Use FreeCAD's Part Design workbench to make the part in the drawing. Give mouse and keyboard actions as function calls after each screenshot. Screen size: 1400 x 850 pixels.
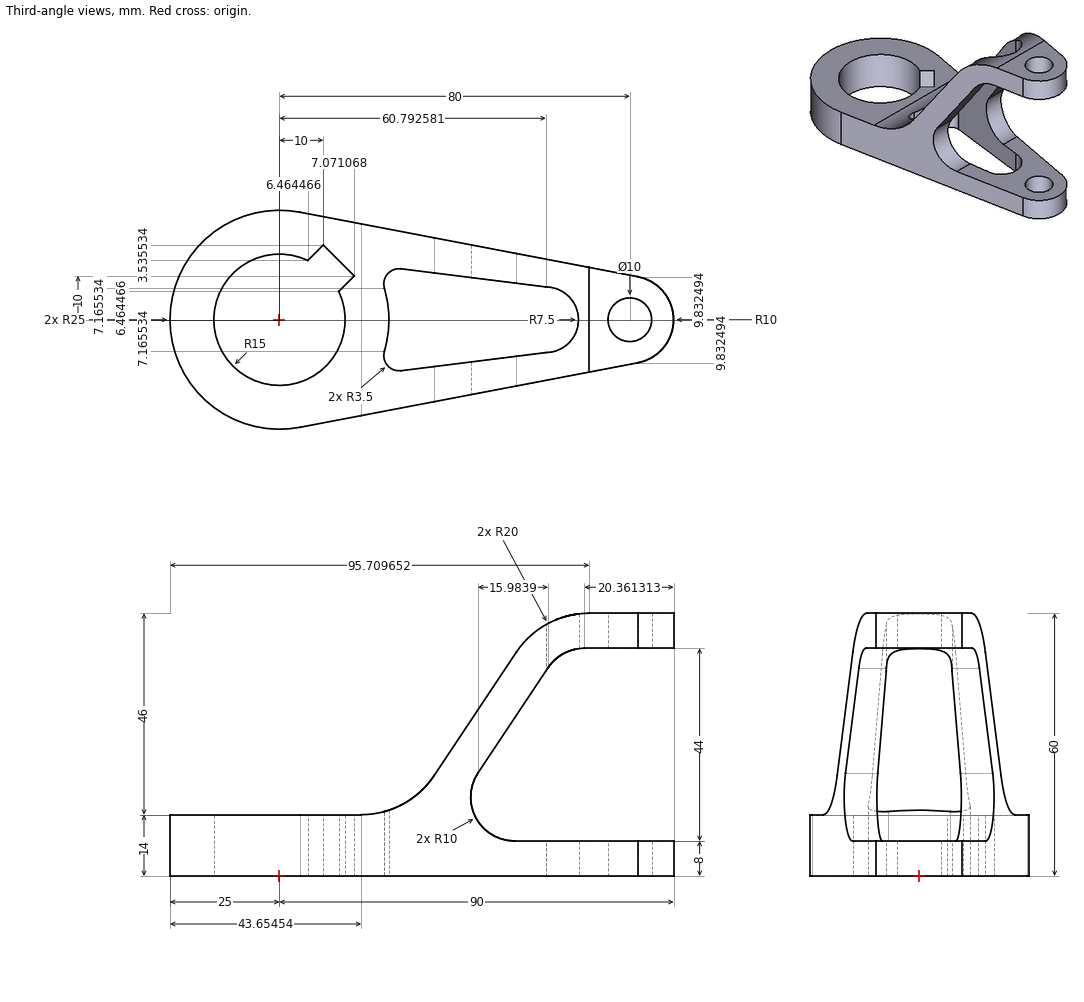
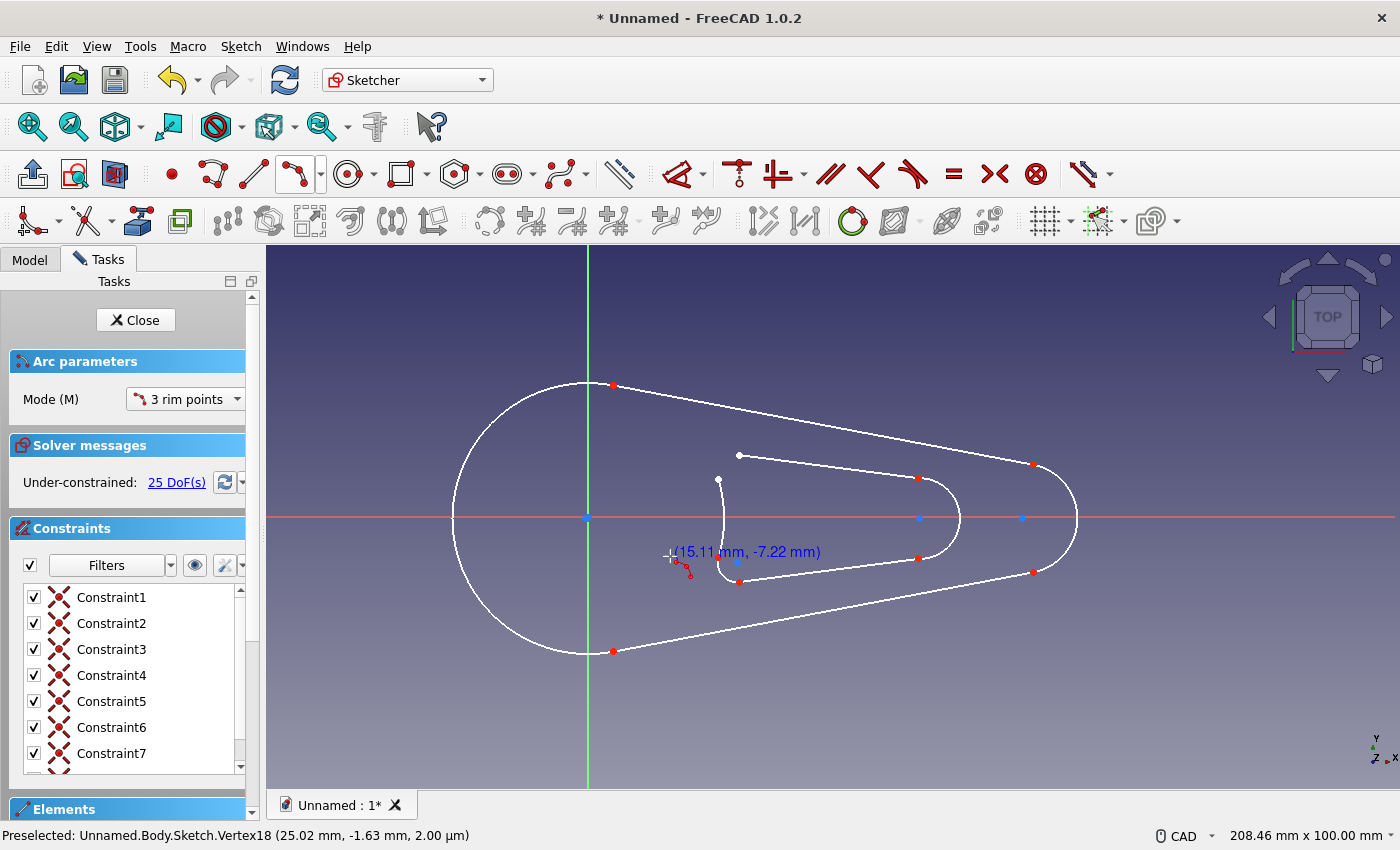
click(718, 479)
click(739, 455)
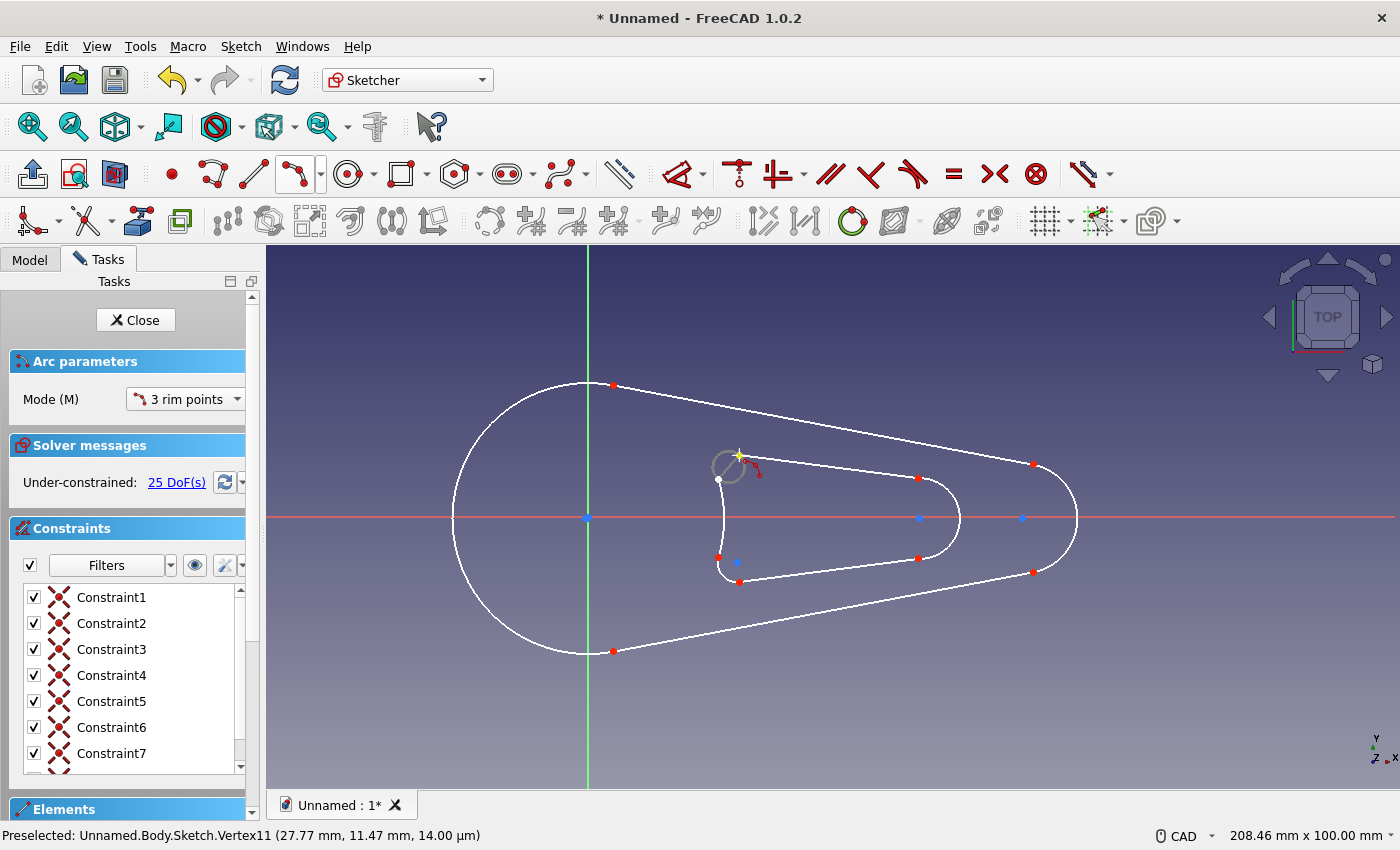
scroll(722, 461, up, 4)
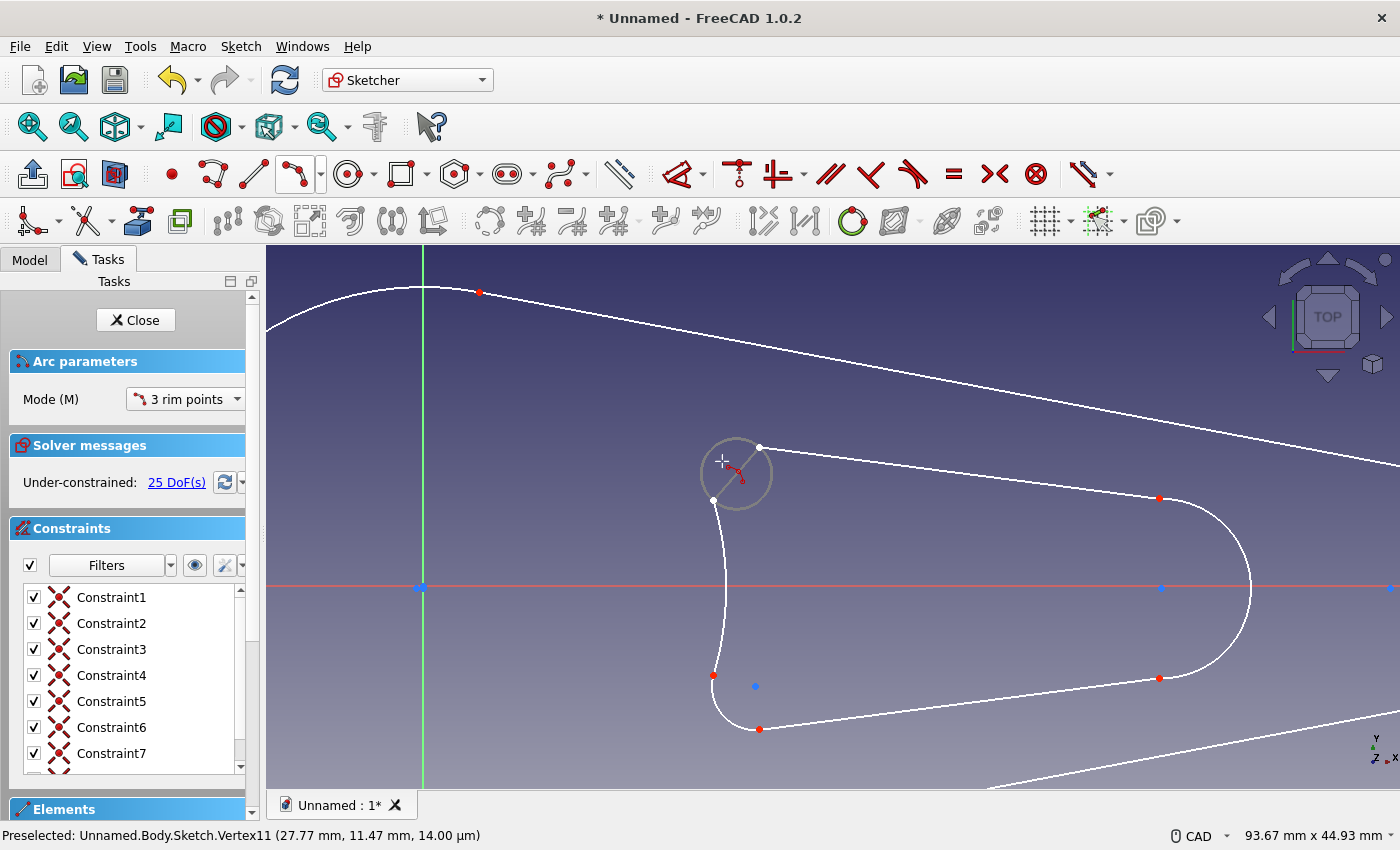
click(722, 460)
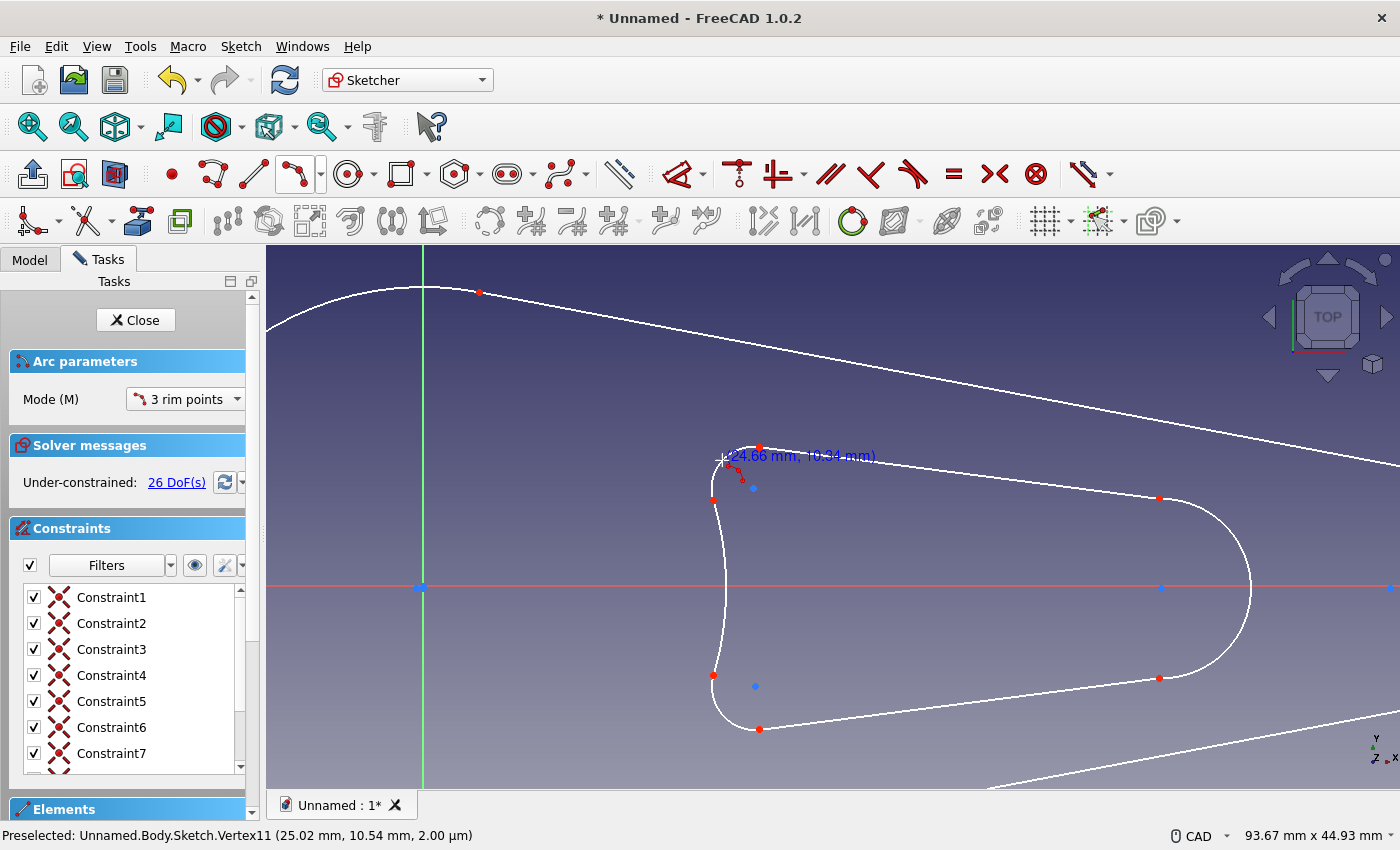
click(213, 174)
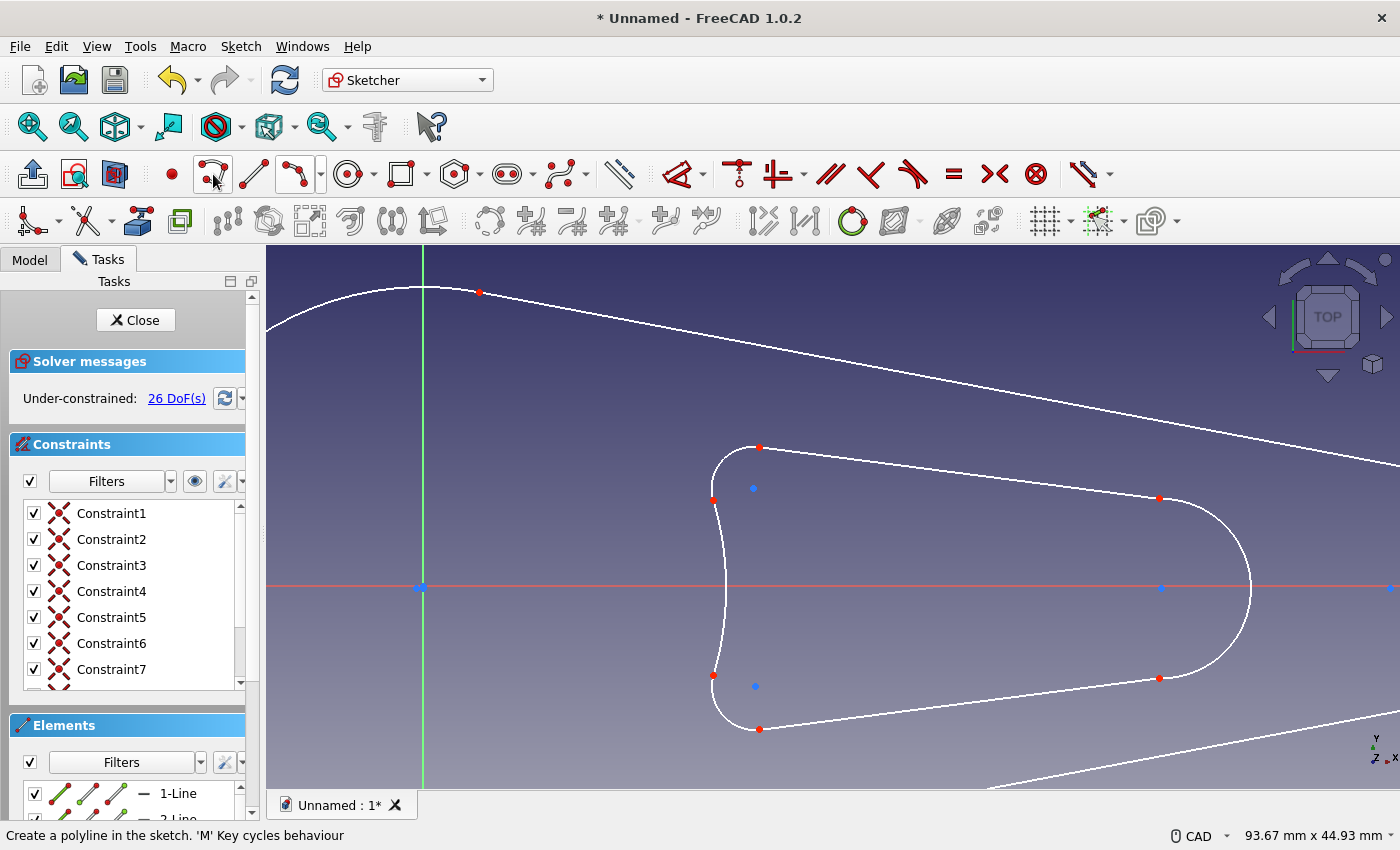
click(502, 422)
click(544, 379)
click(630, 465)
click(587, 508)
right_click(587, 508)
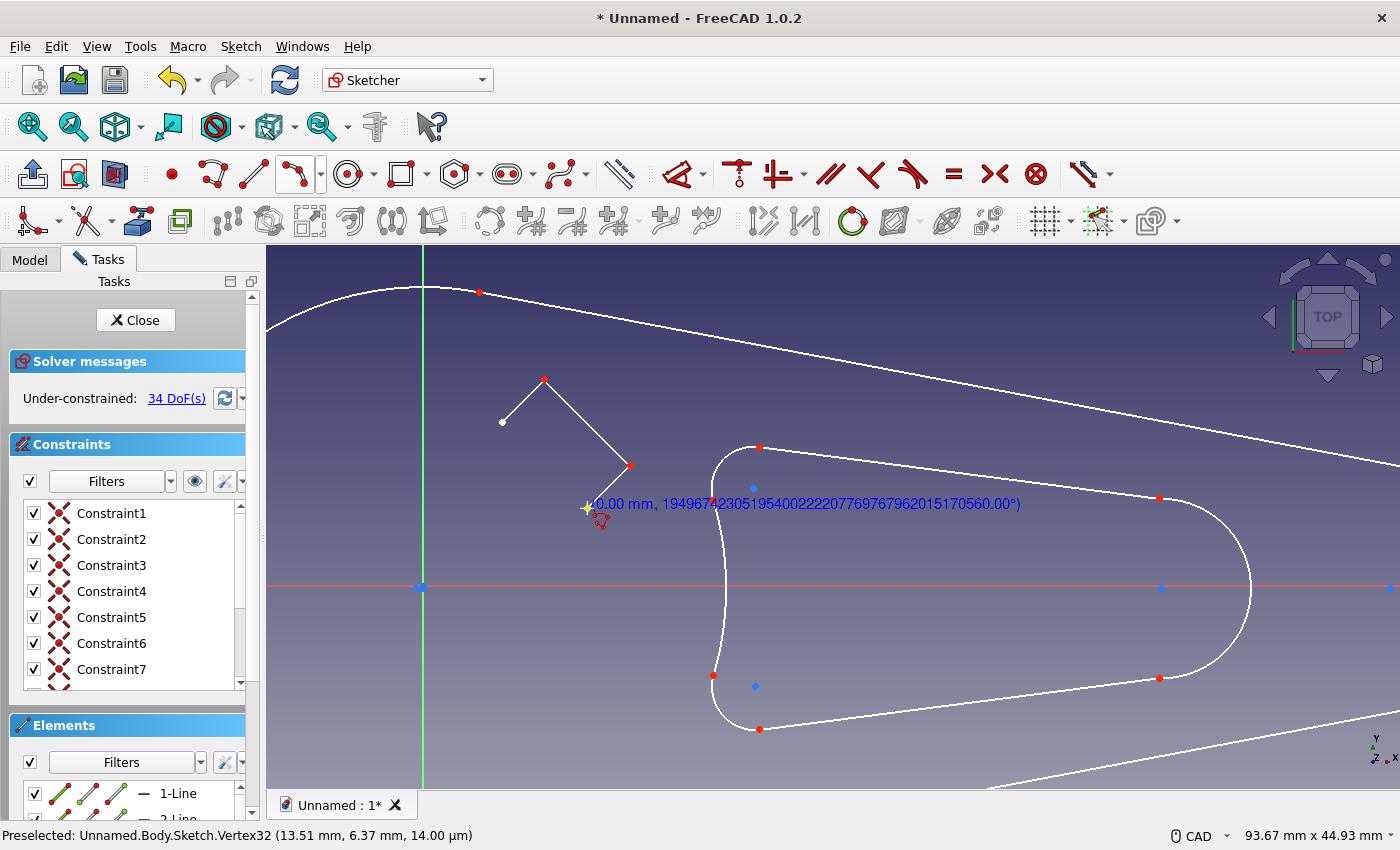
click(294, 174)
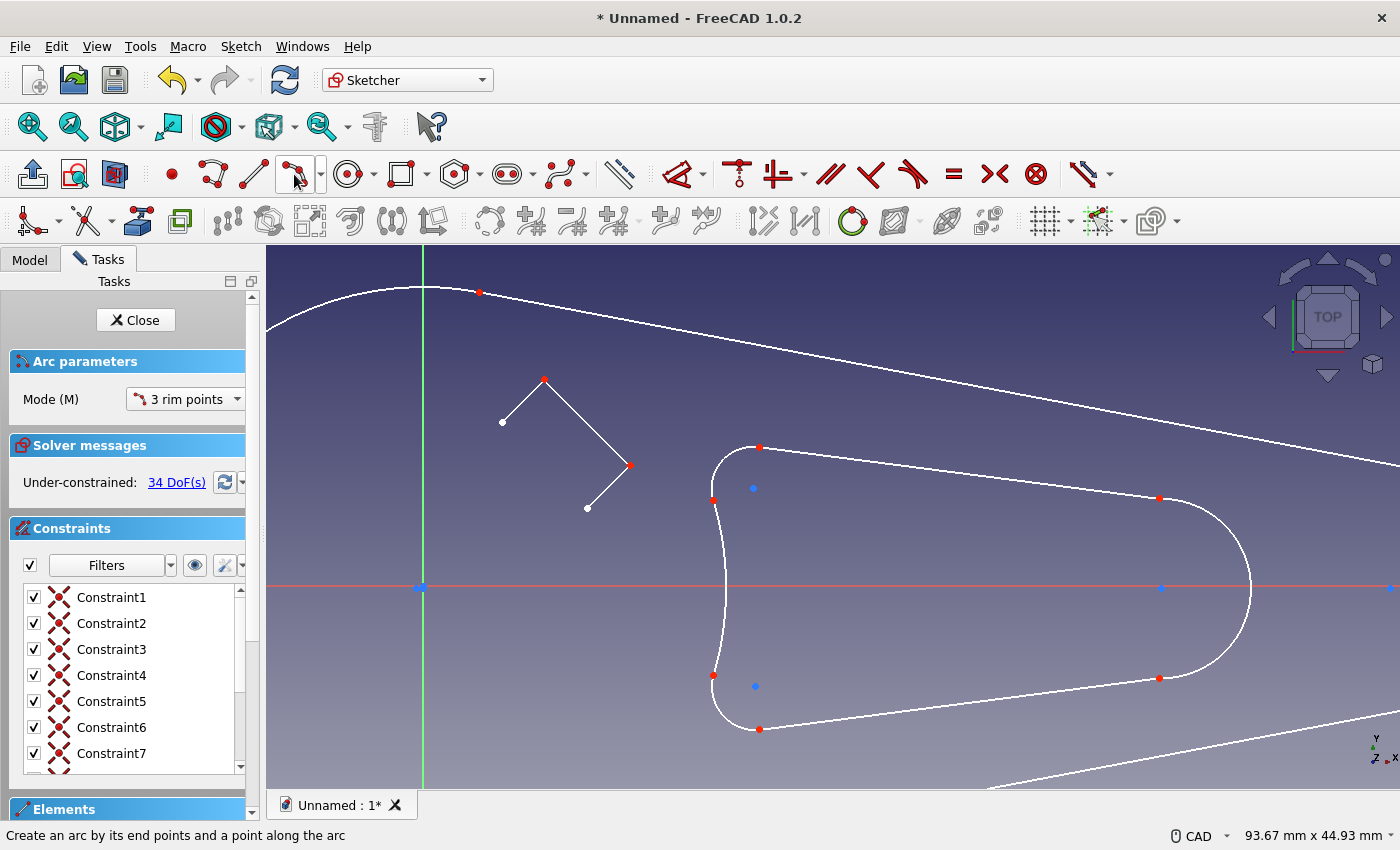
click(587, 509)
click(502, 423)
click(295, 715)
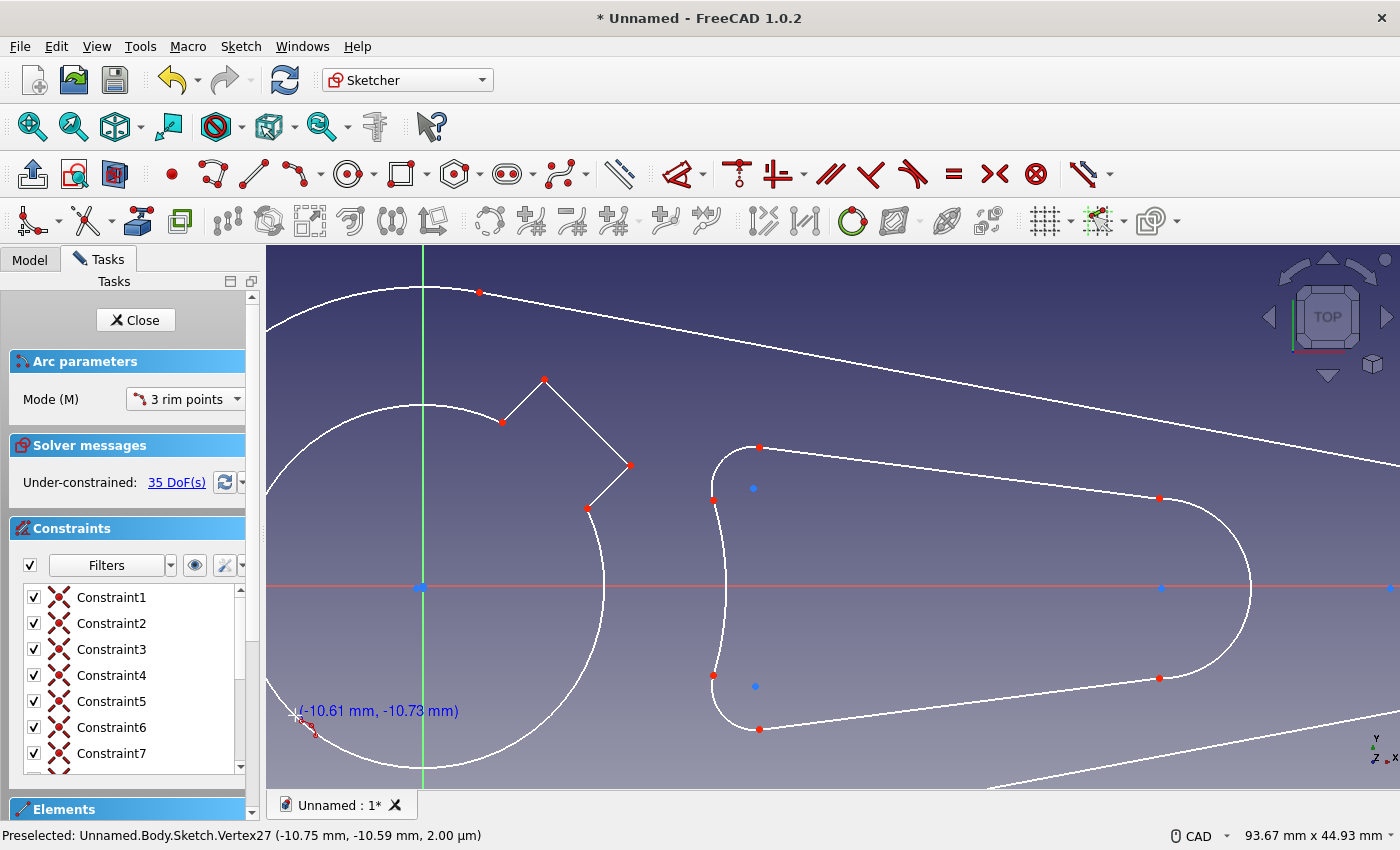
key(g)
key(c)